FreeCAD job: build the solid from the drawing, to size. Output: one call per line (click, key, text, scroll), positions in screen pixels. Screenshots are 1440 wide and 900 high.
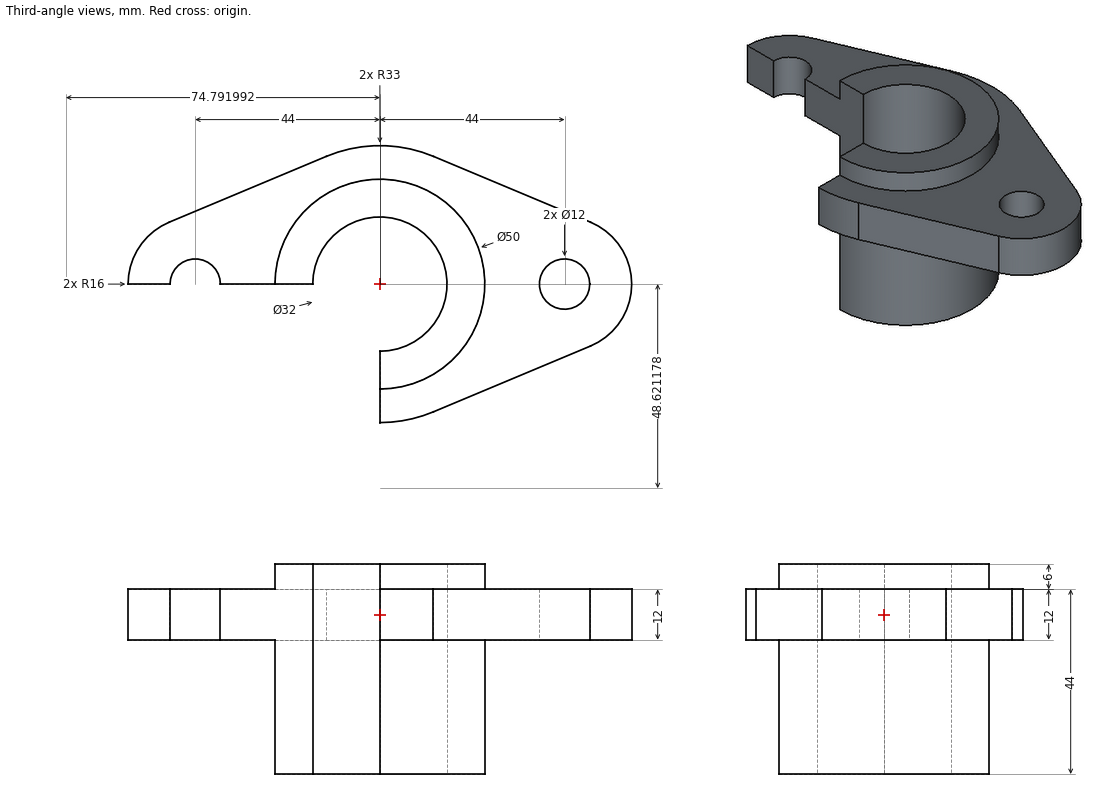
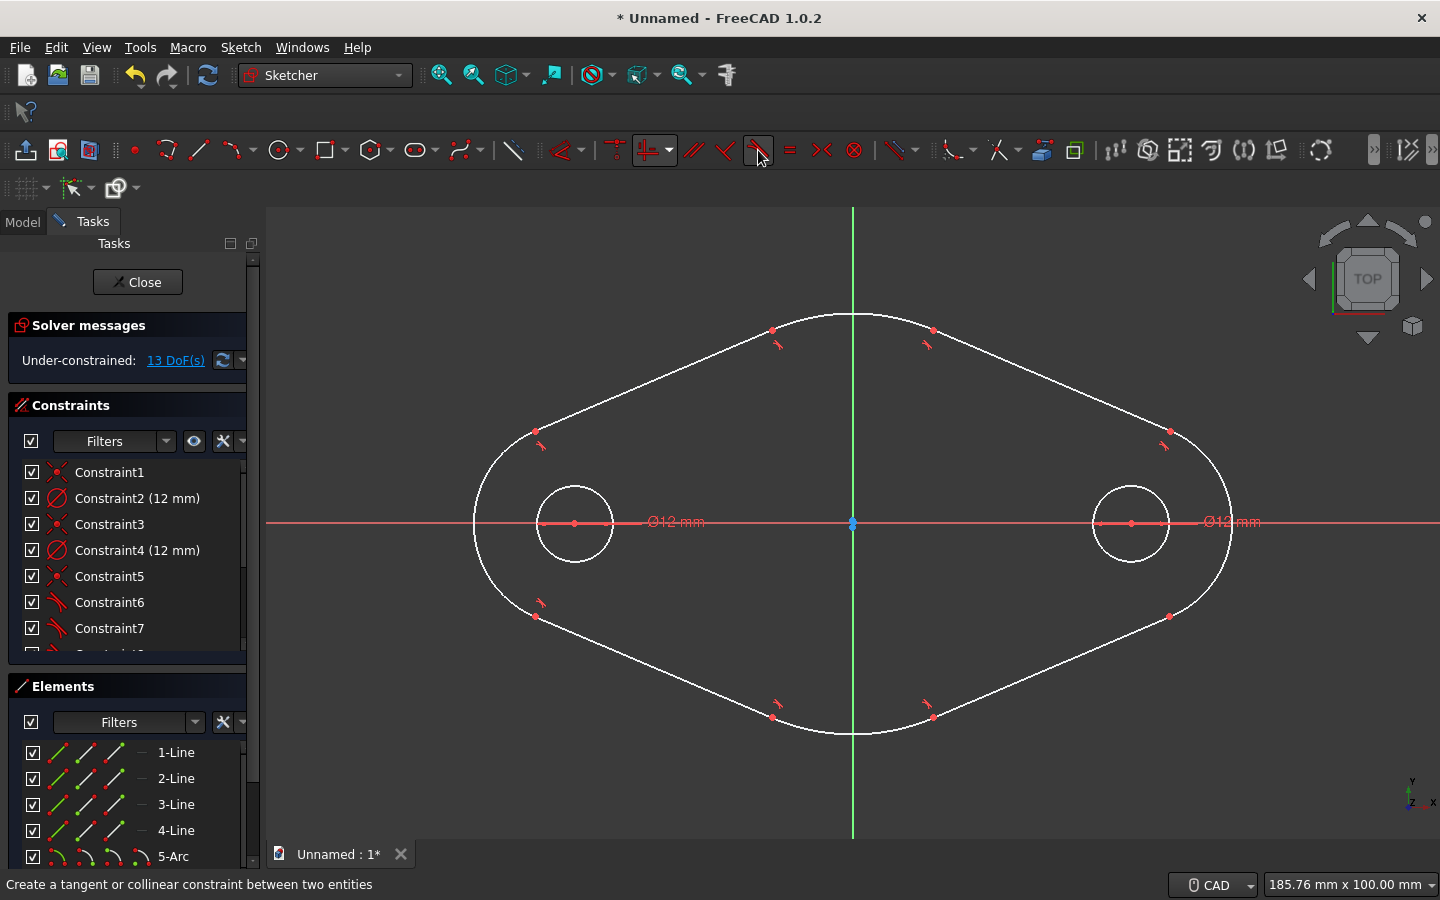
click(1005, 688)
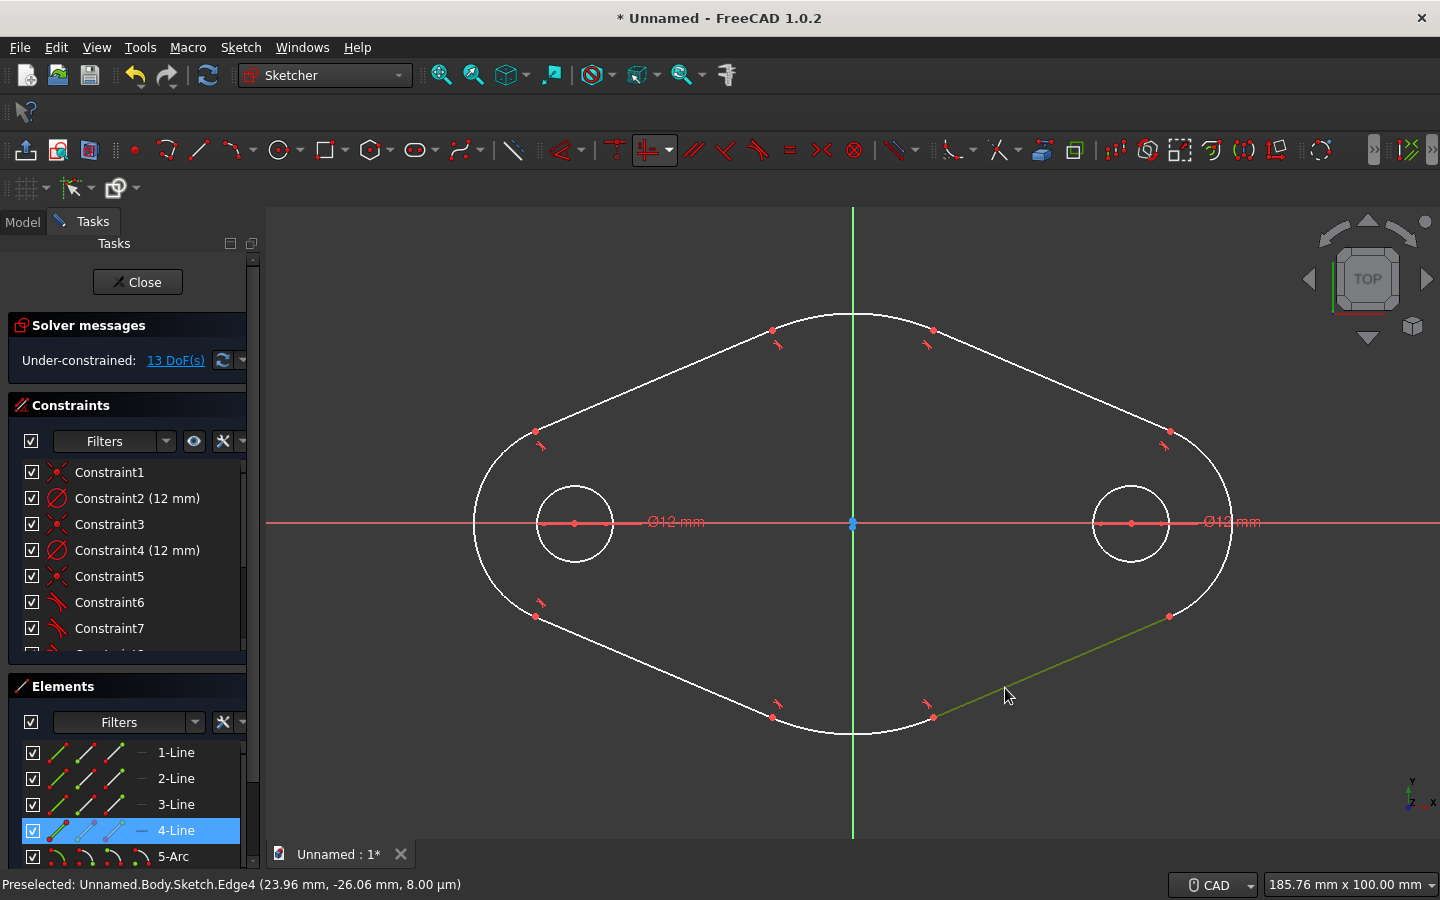
click(1221, 570)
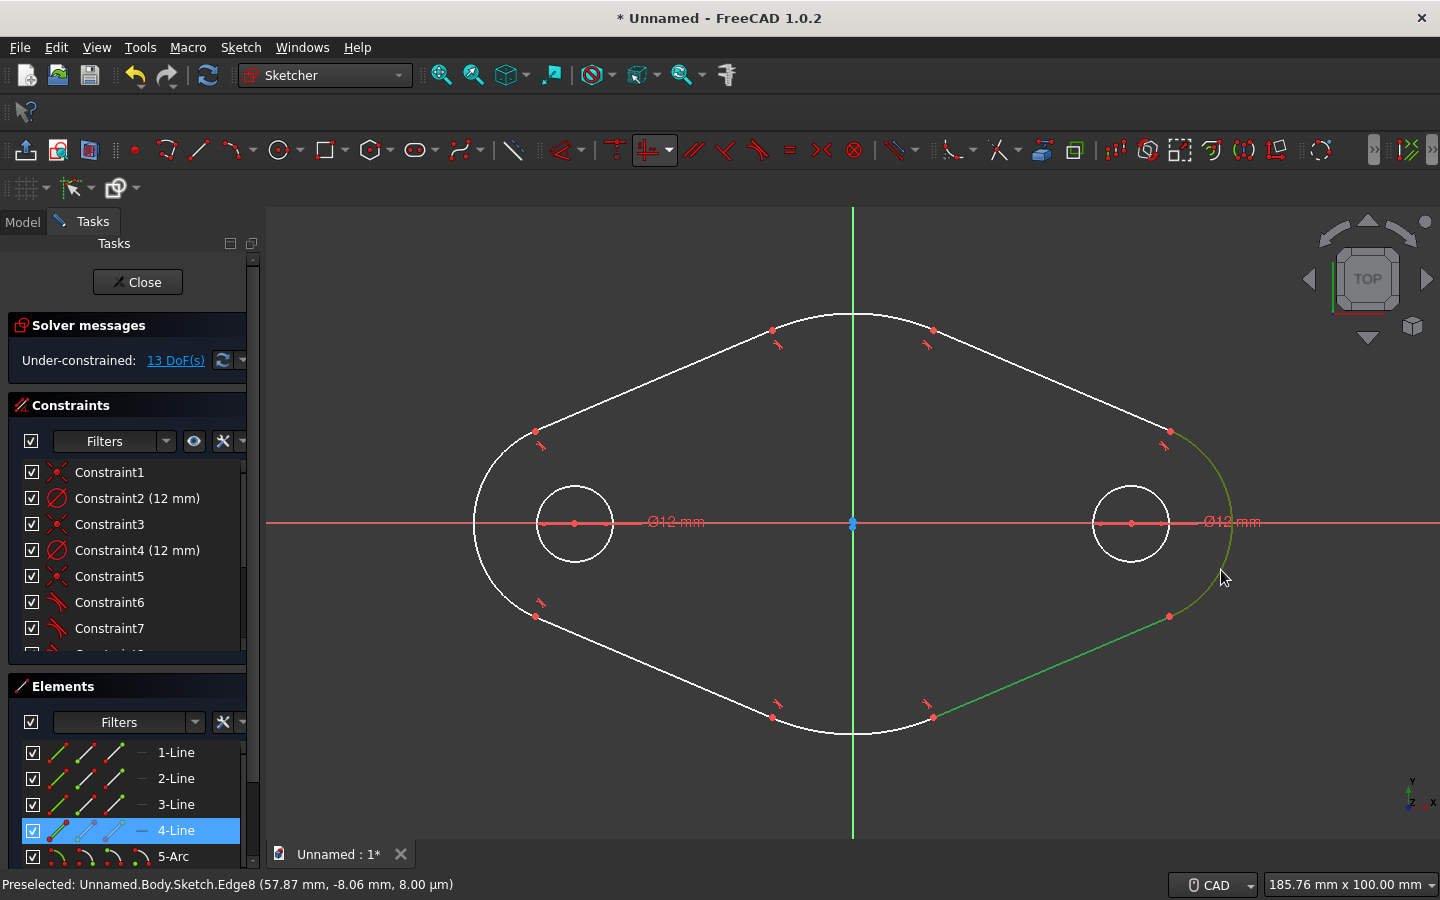
click(758, 150)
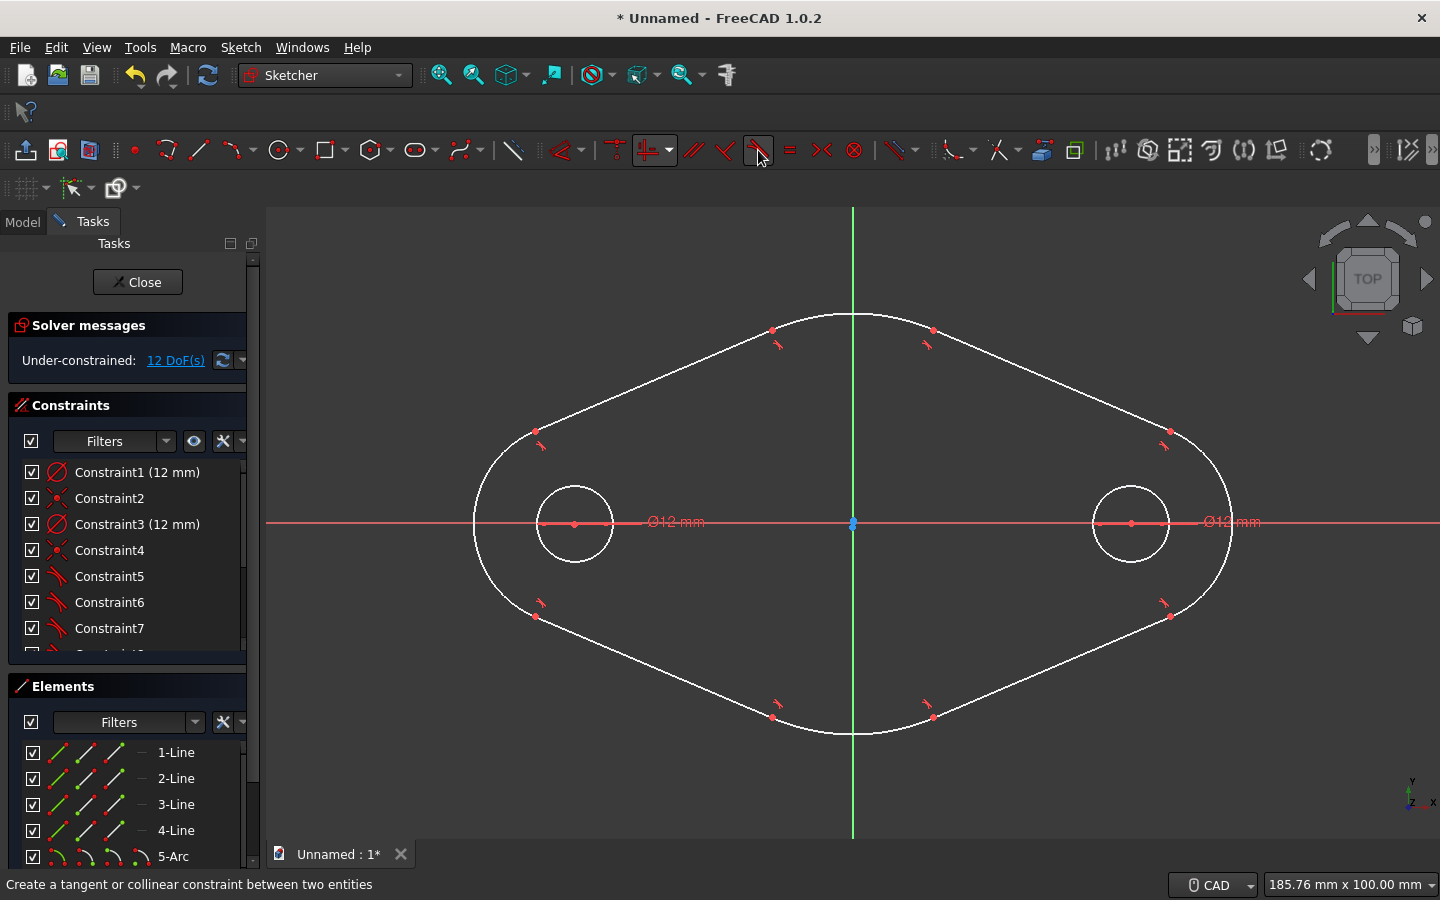
click(886, 316)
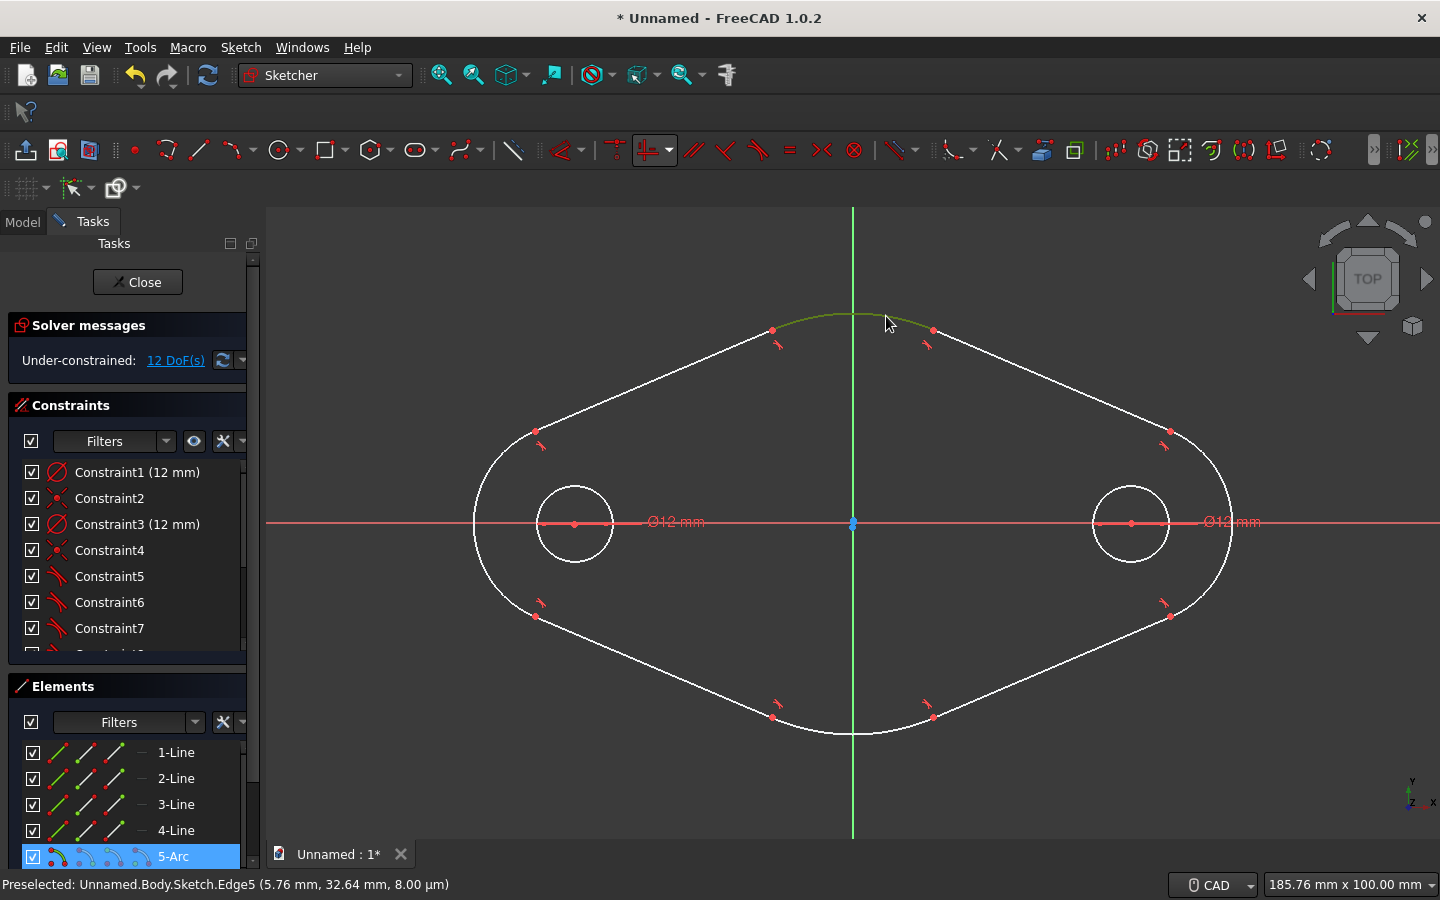
click(820, 732)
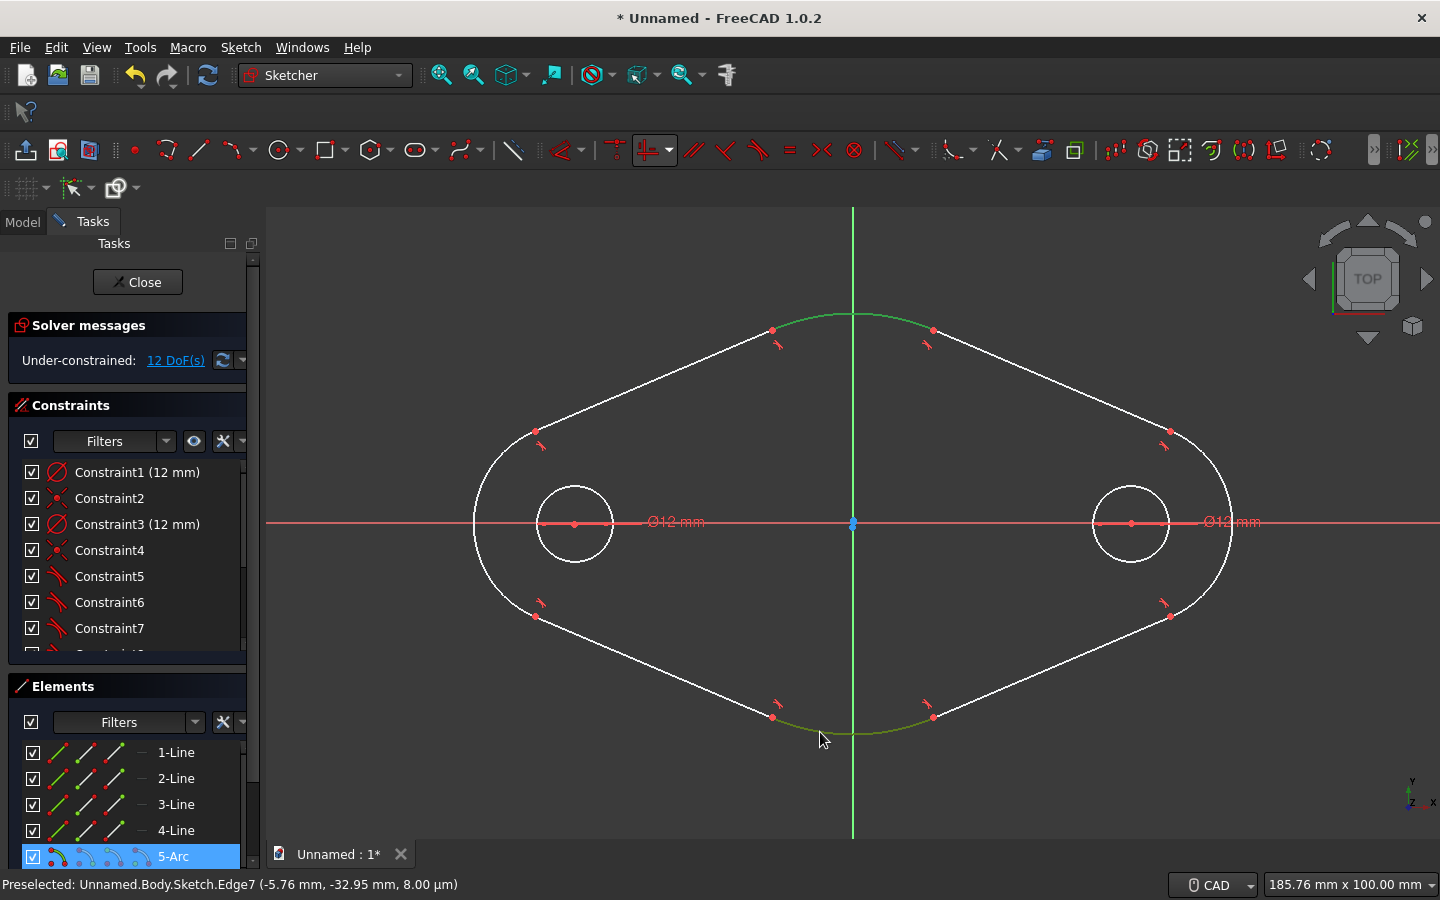
click(616, 150)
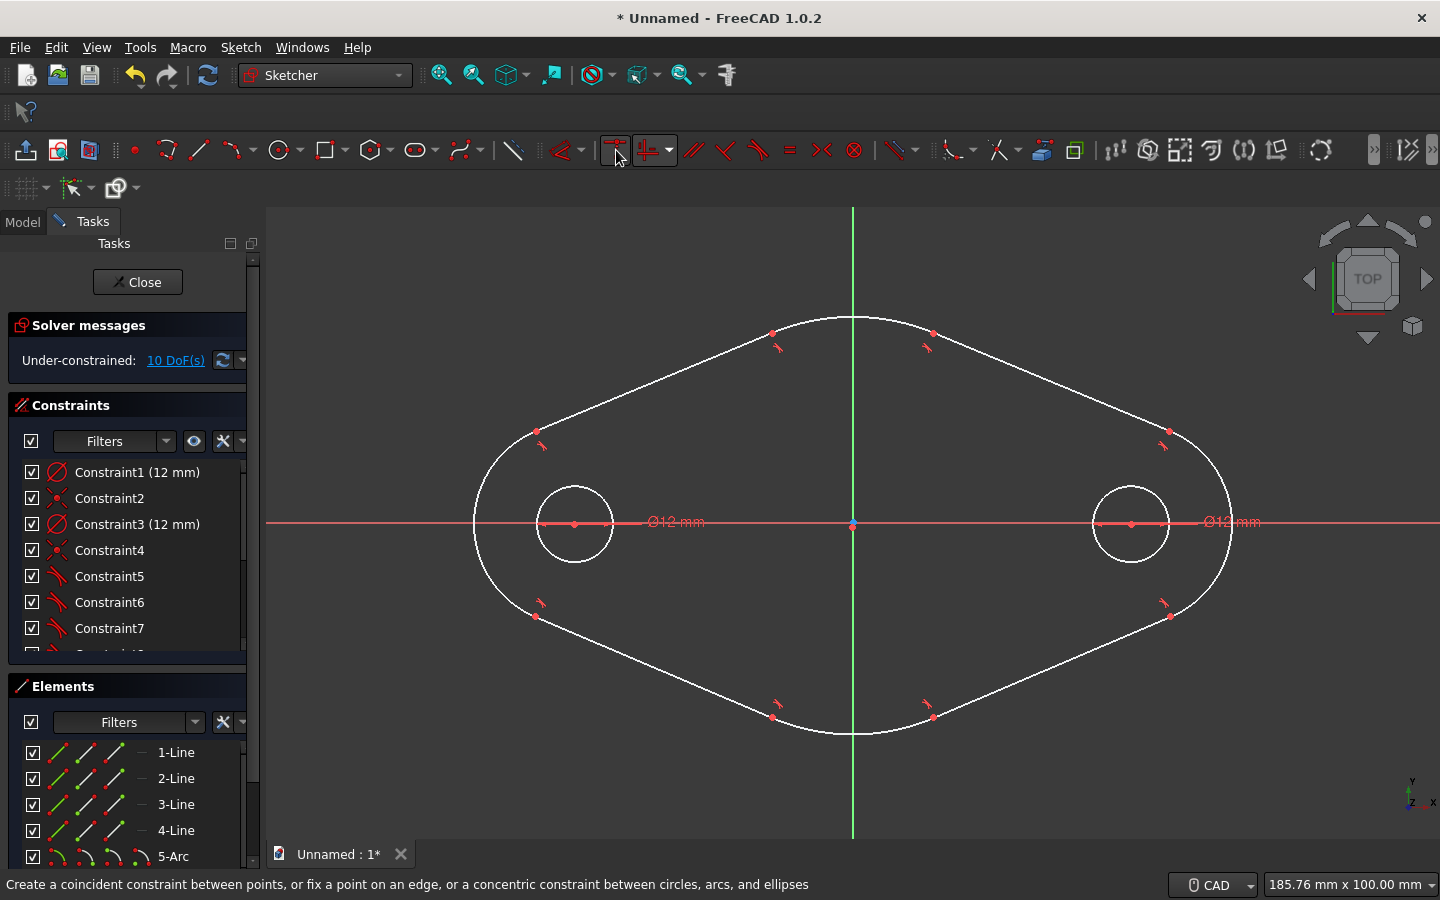
drag(843, 513, 863, 538)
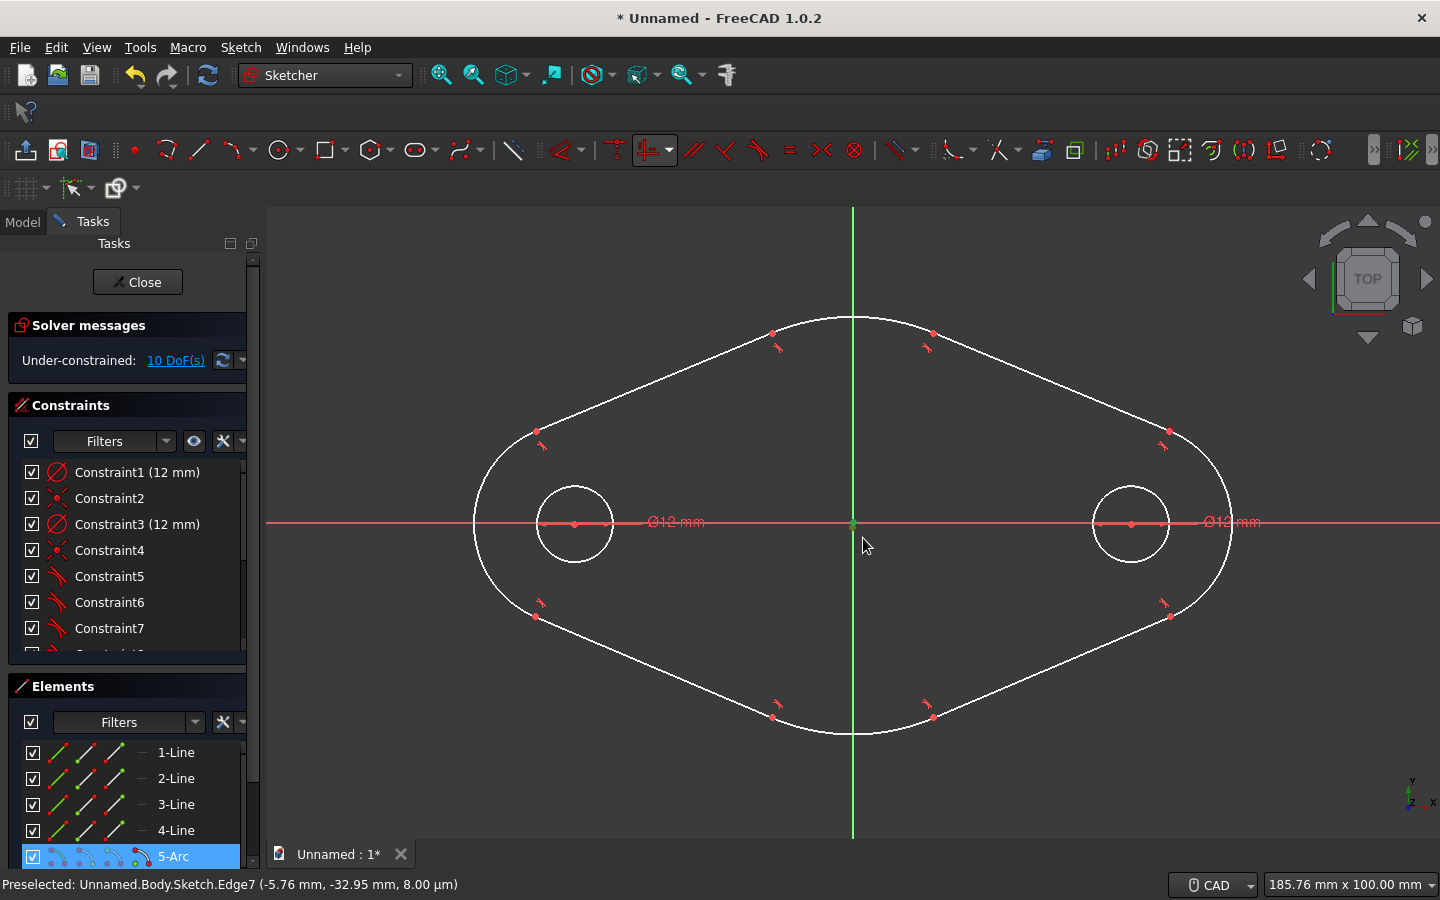
click(616, 150)